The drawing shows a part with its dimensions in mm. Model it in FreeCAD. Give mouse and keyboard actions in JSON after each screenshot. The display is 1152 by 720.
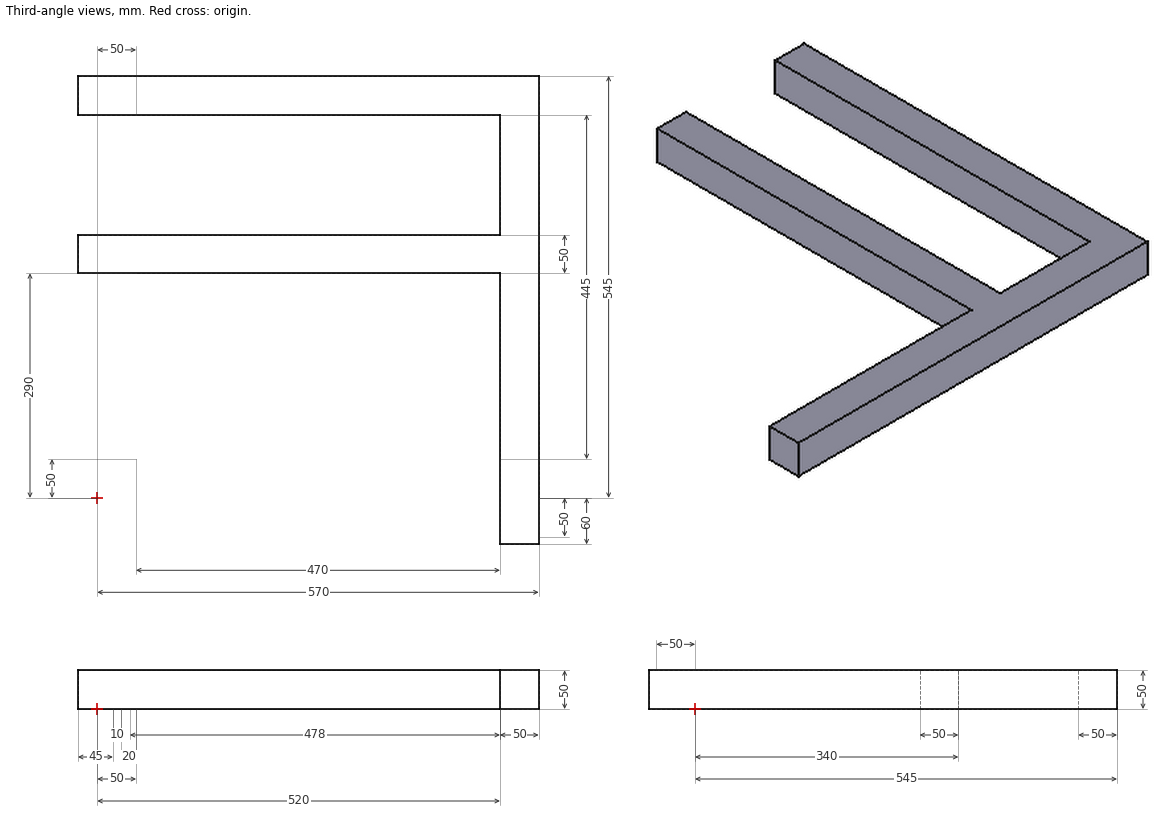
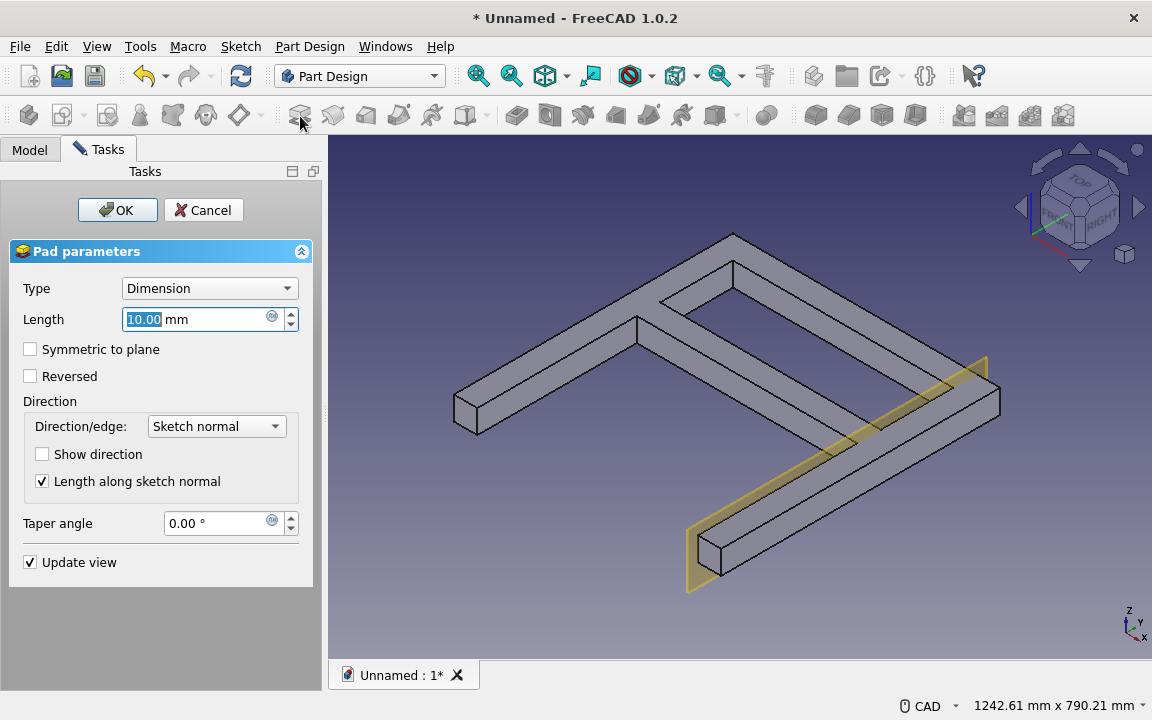
{"action": "type", "text": "478"}
{"action": "key", "text": "Tab"}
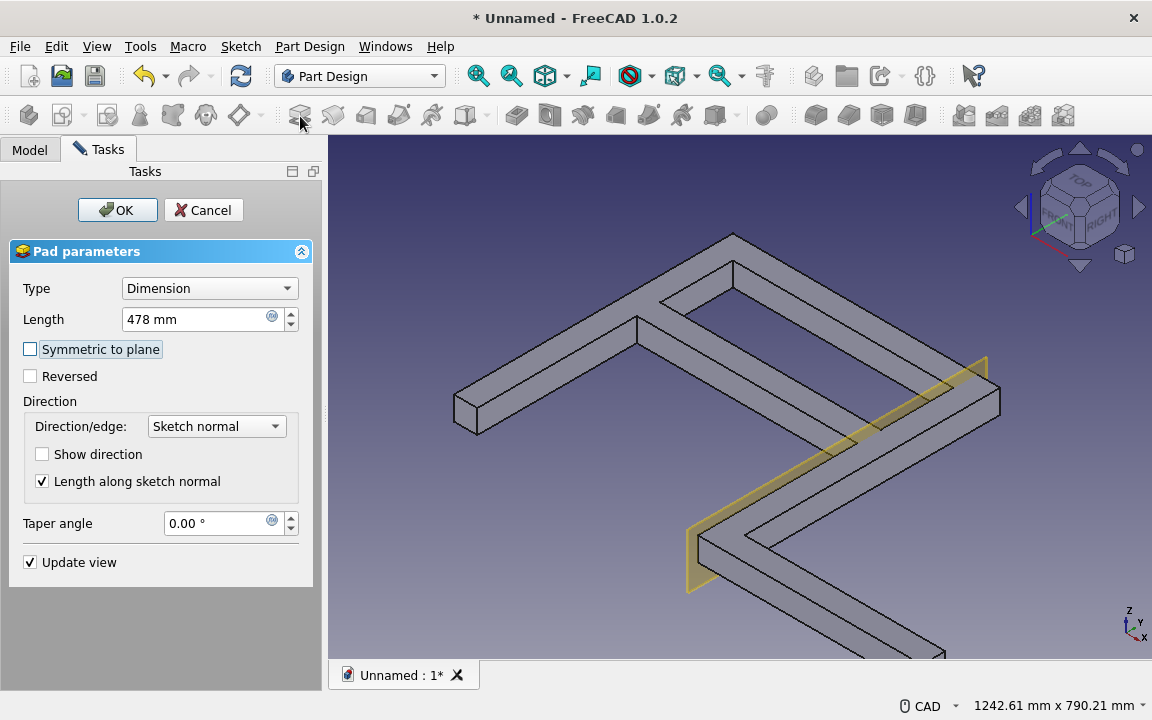
{"action": "left_click", "coordinate": [31, 376]}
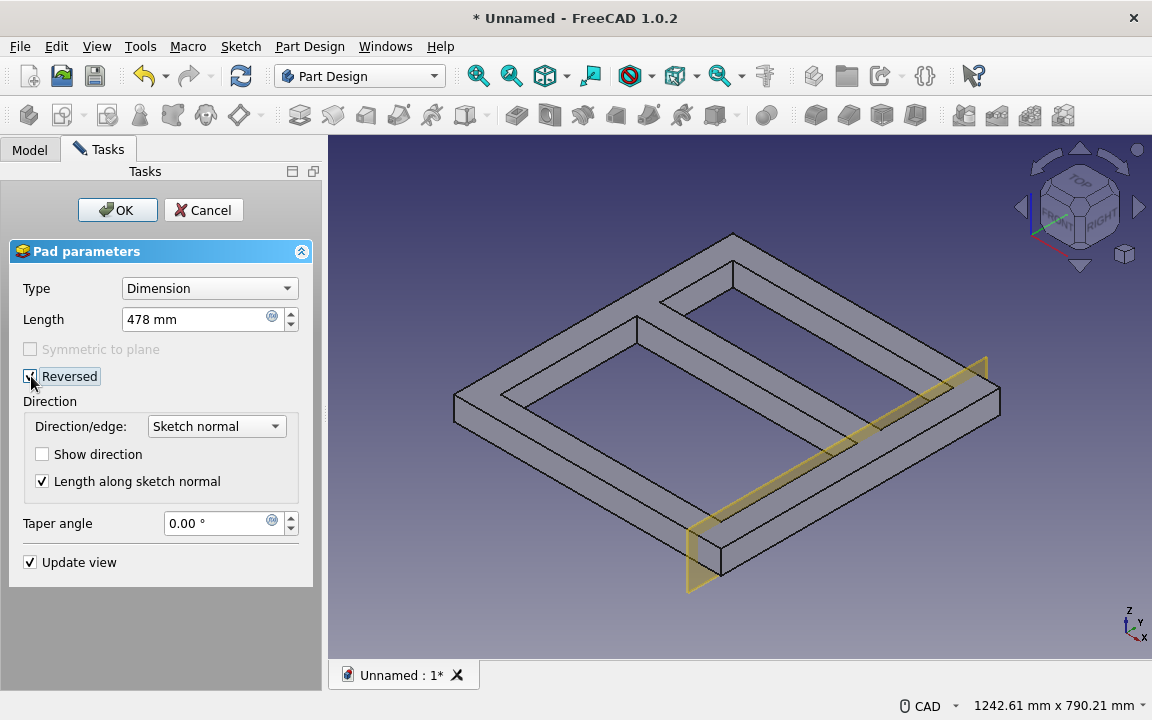
{"action": "left_click", "coordinate": [118, 210]}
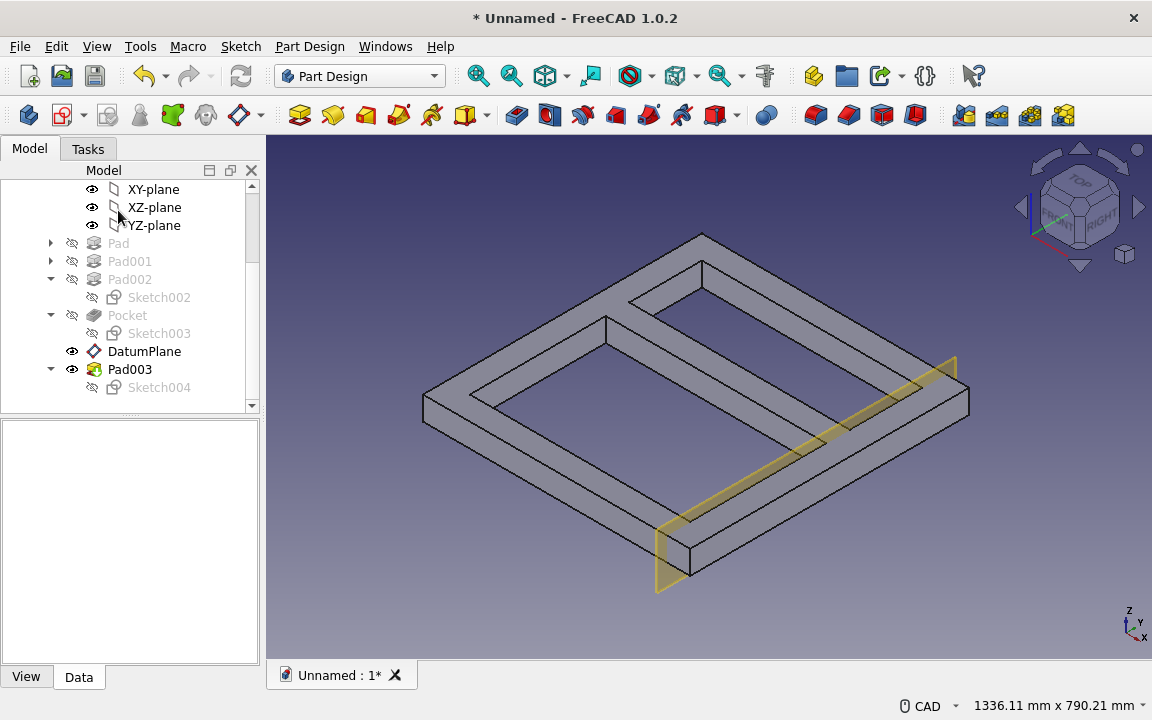
{"action": "left_click", "coordinate": [117, 351]}
{"action": "key", "text": "space"}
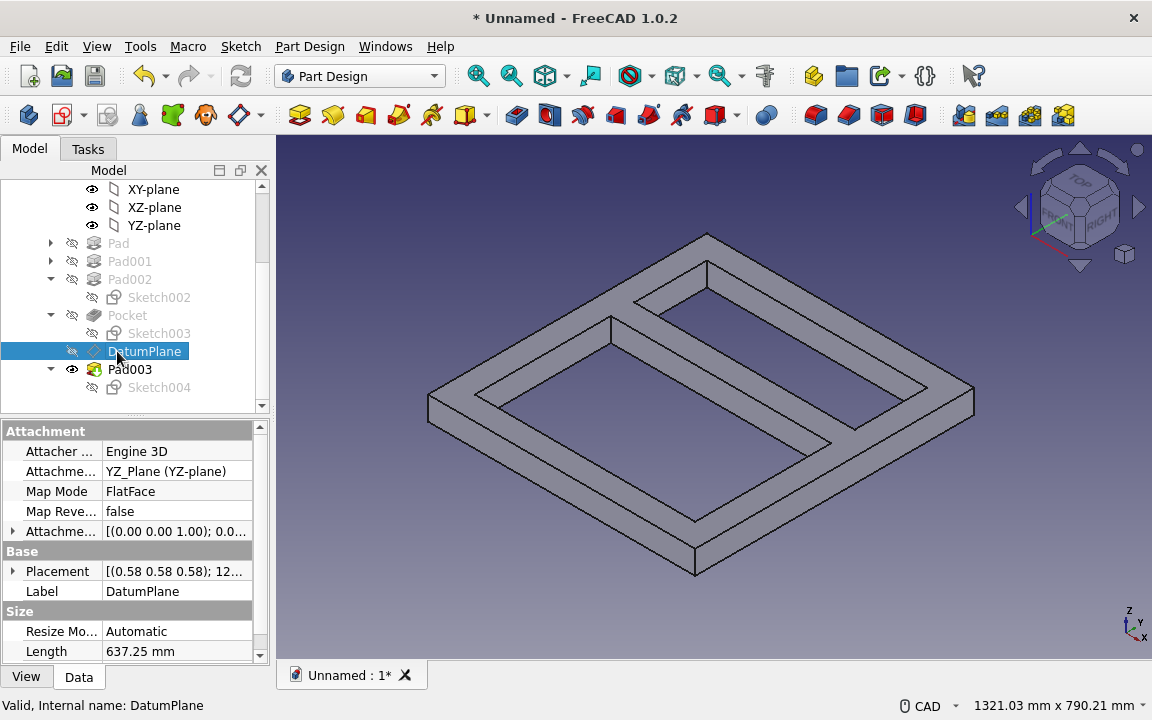
{"action": "left_click", "coordinate": [935, 387]}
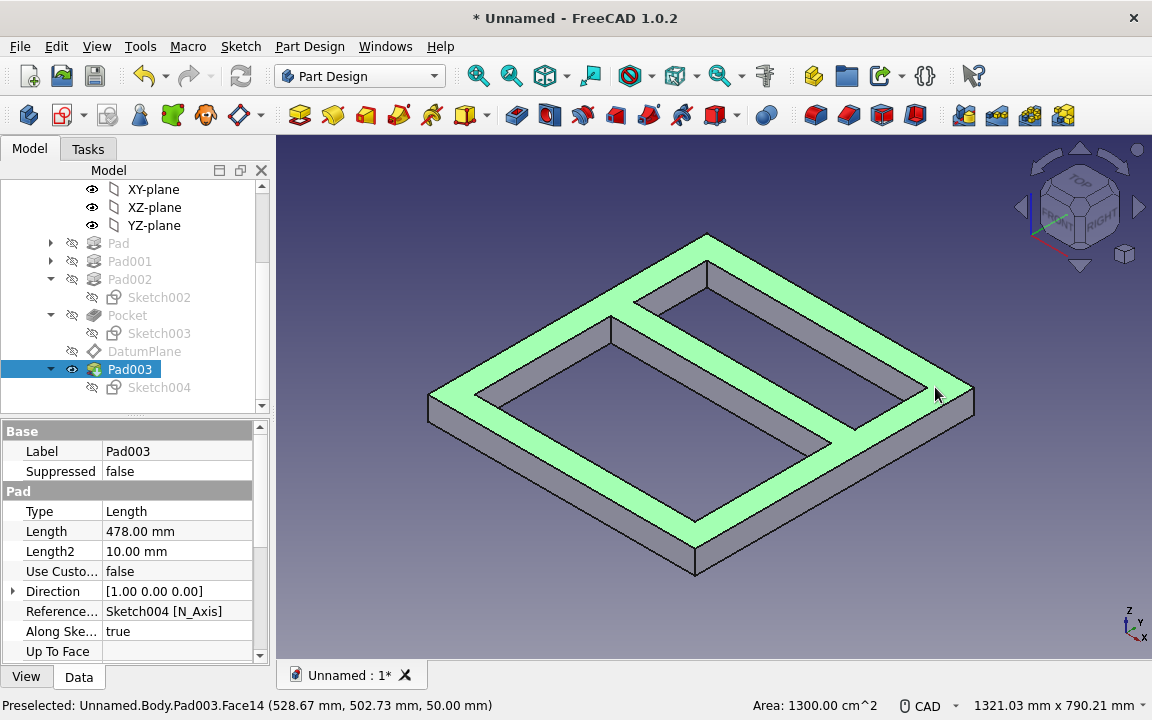
{"action": "left_click", "coordinate": [62, 116]}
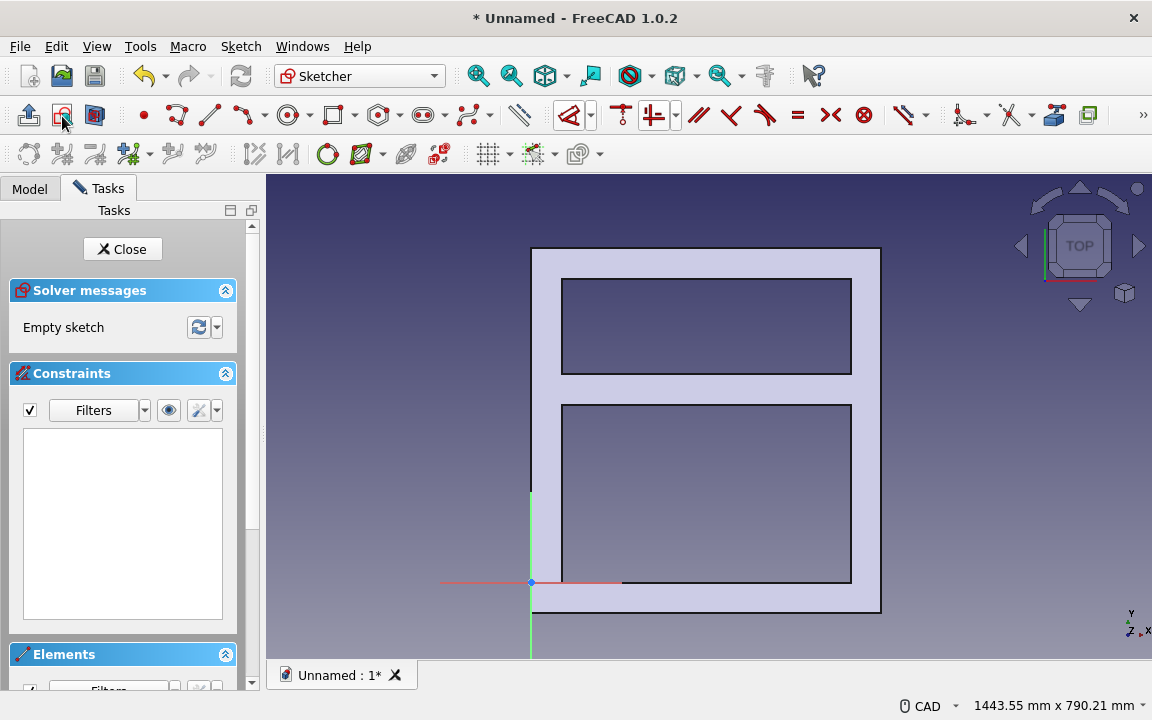
{"action": "scroll", "coordinate": [840, 631], "scroll_direction": "up", "scroll_amount": 2}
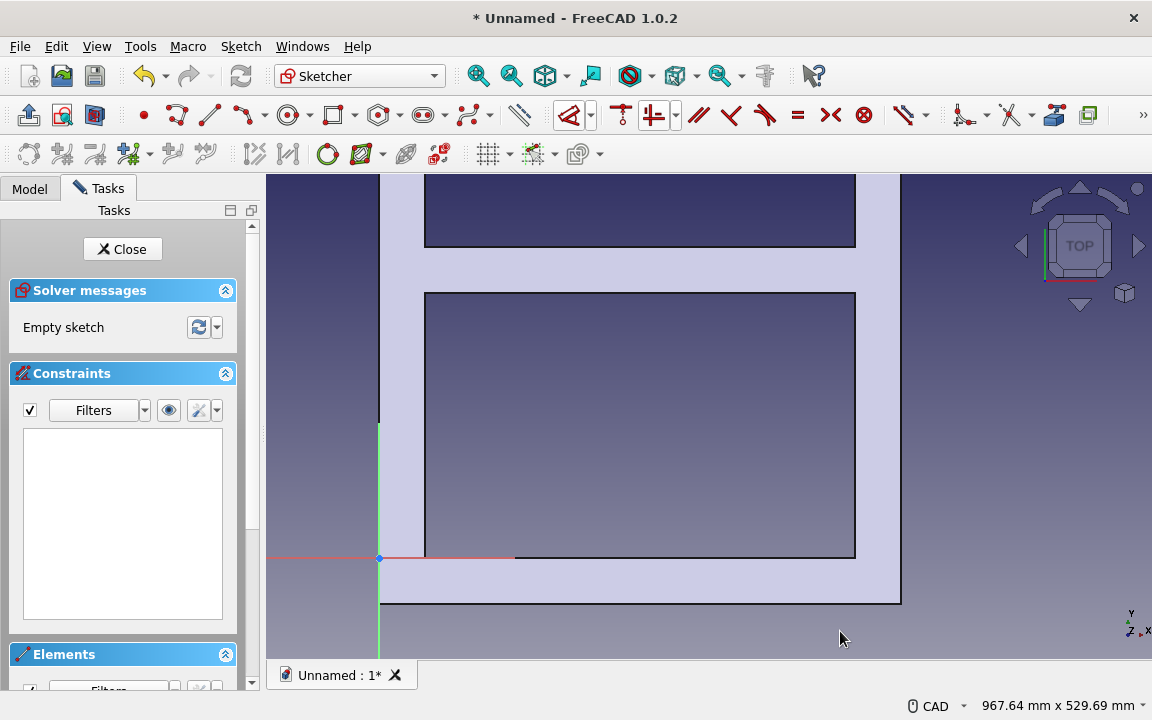
{"action": "key", "text": "g r"}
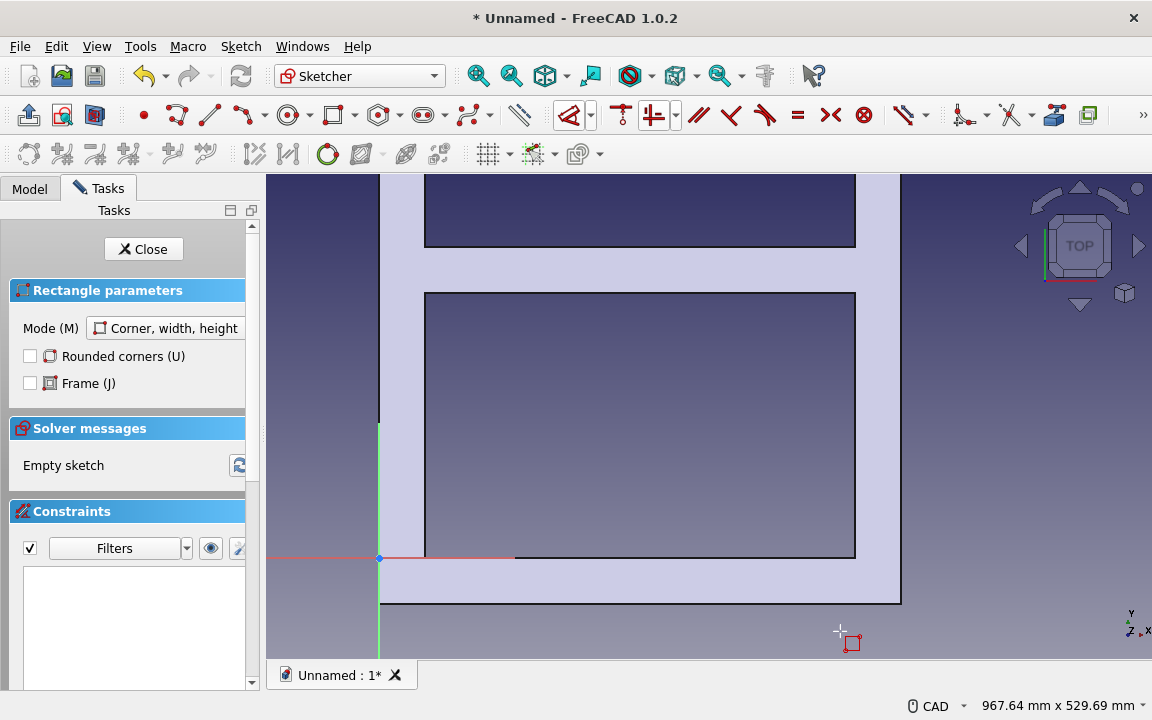
{"action": "left_click", "coordinate": [379, 558]}
{"action": "mouse_move", "coordinate": [901, 604]}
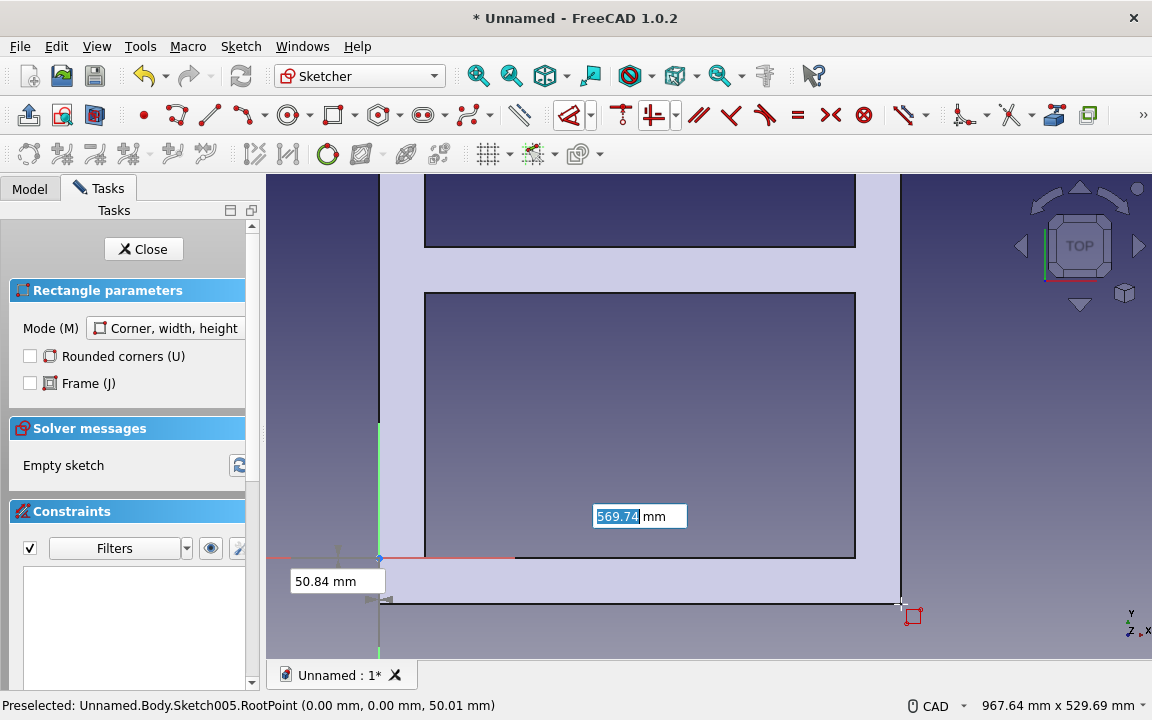
{"action": "type", "text": "570"}
{"action": "key", "text": "Tab"}
{"action": "type", "text": "50"}
{"action": "key", "text": "Return"}
{"action": "key", "text": "Escape"}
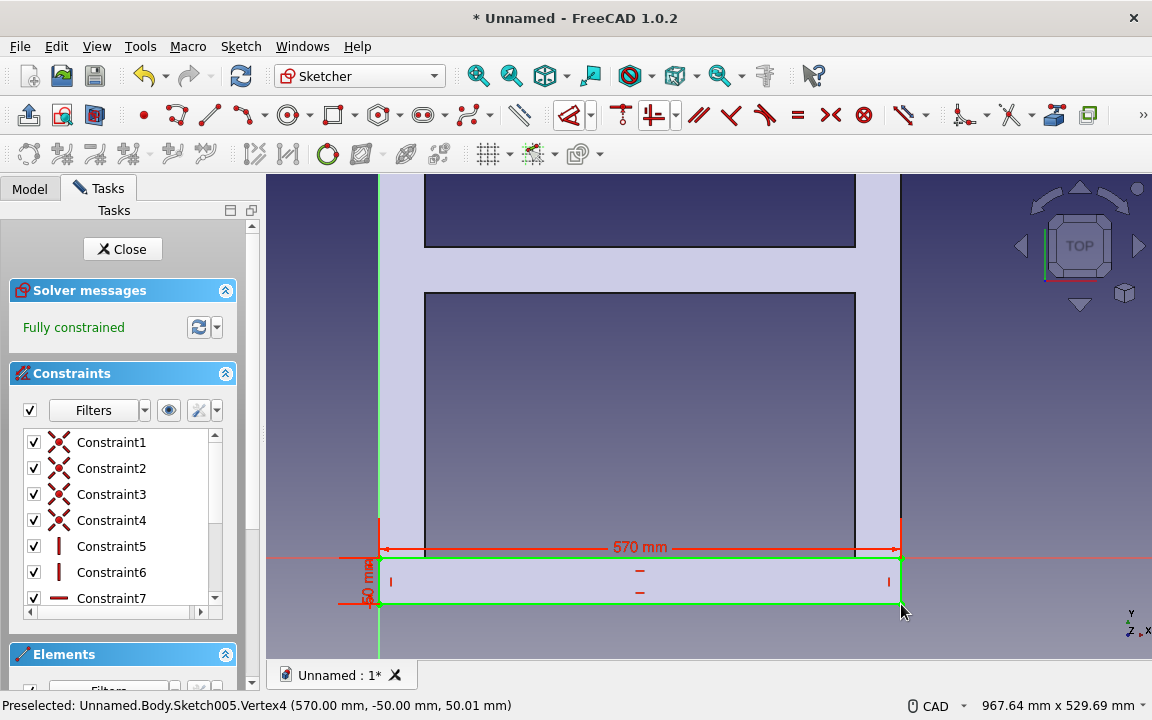
{"action": "left_click", "coordinate": [123, 249]}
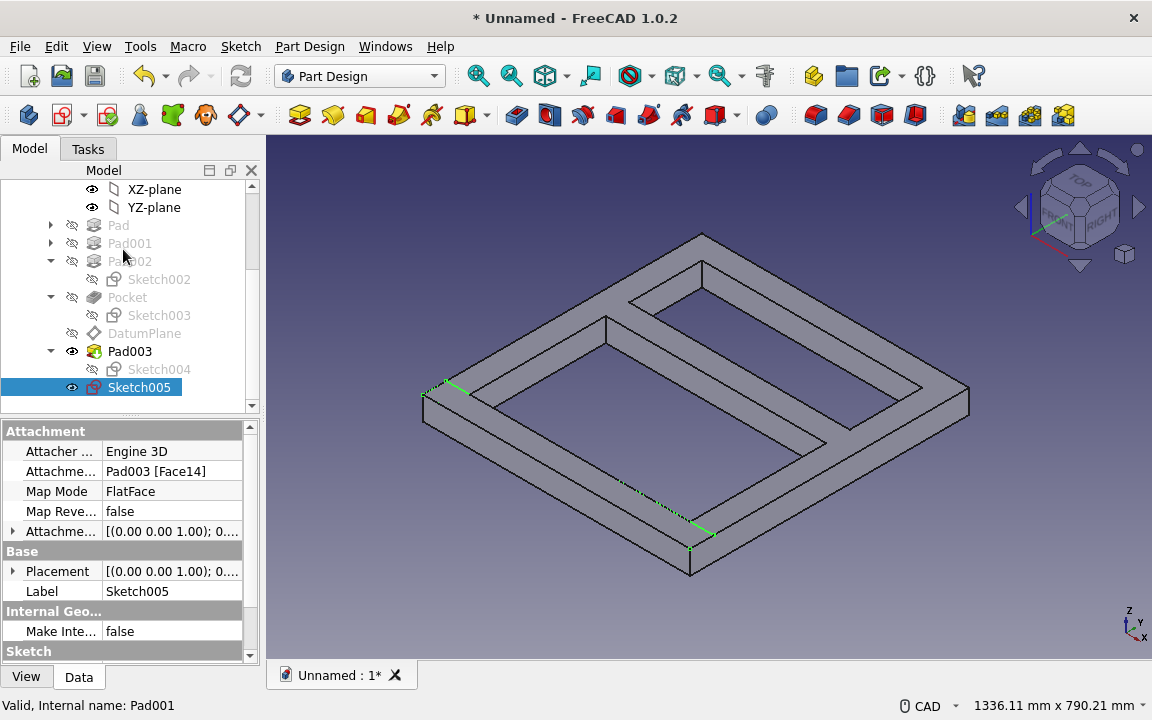
{"action": "left_click", "coordinate": [517, 116]}